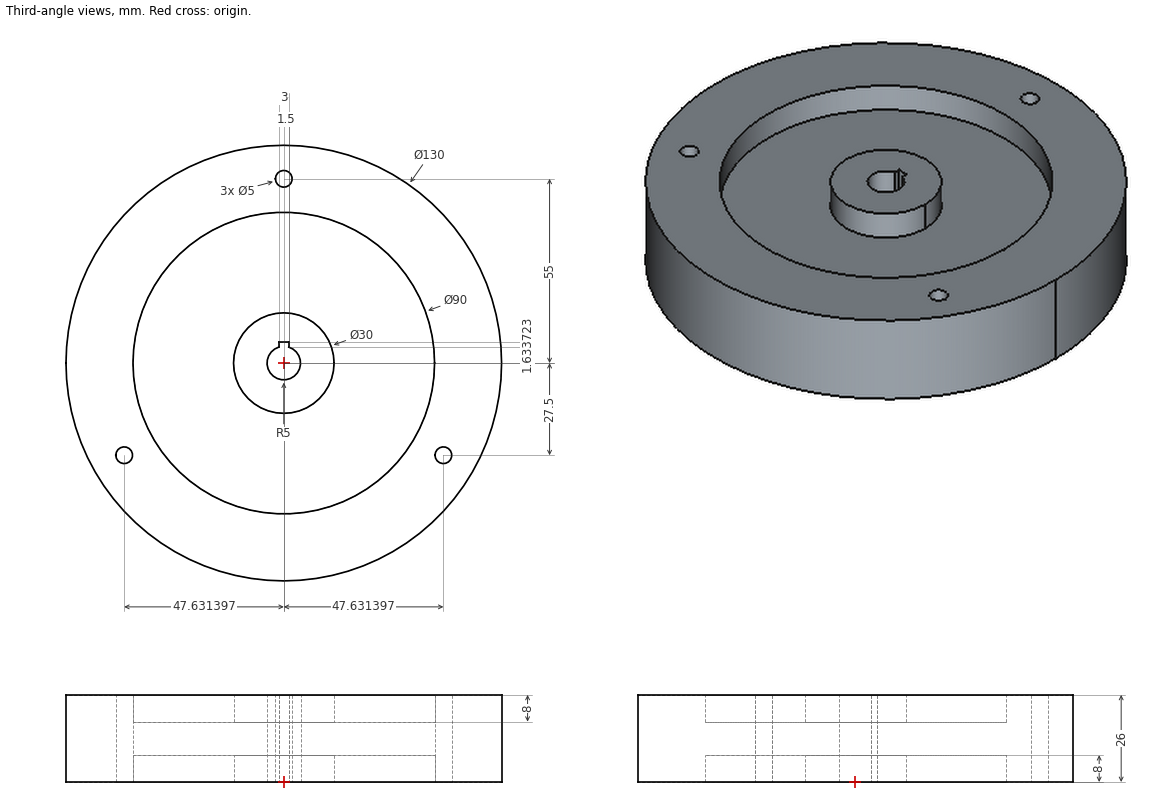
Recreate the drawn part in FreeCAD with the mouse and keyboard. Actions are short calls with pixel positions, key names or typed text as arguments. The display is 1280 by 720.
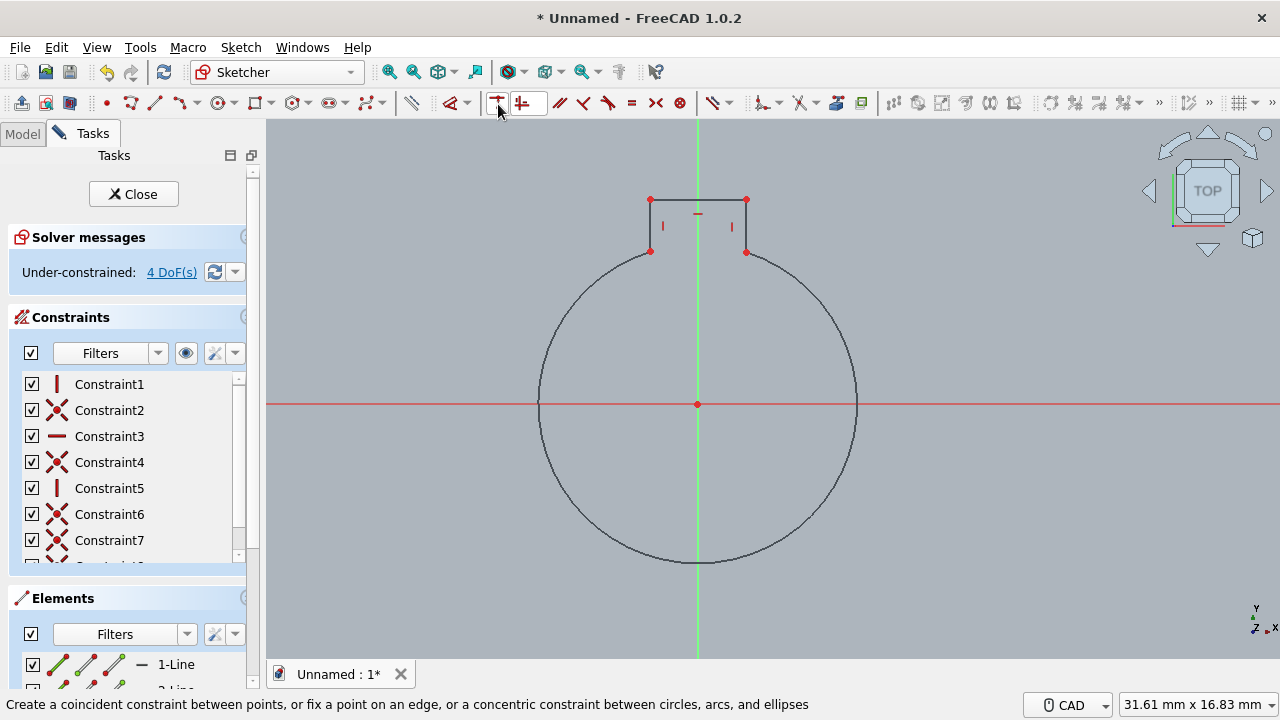
click(553, 471)
click(524, 484)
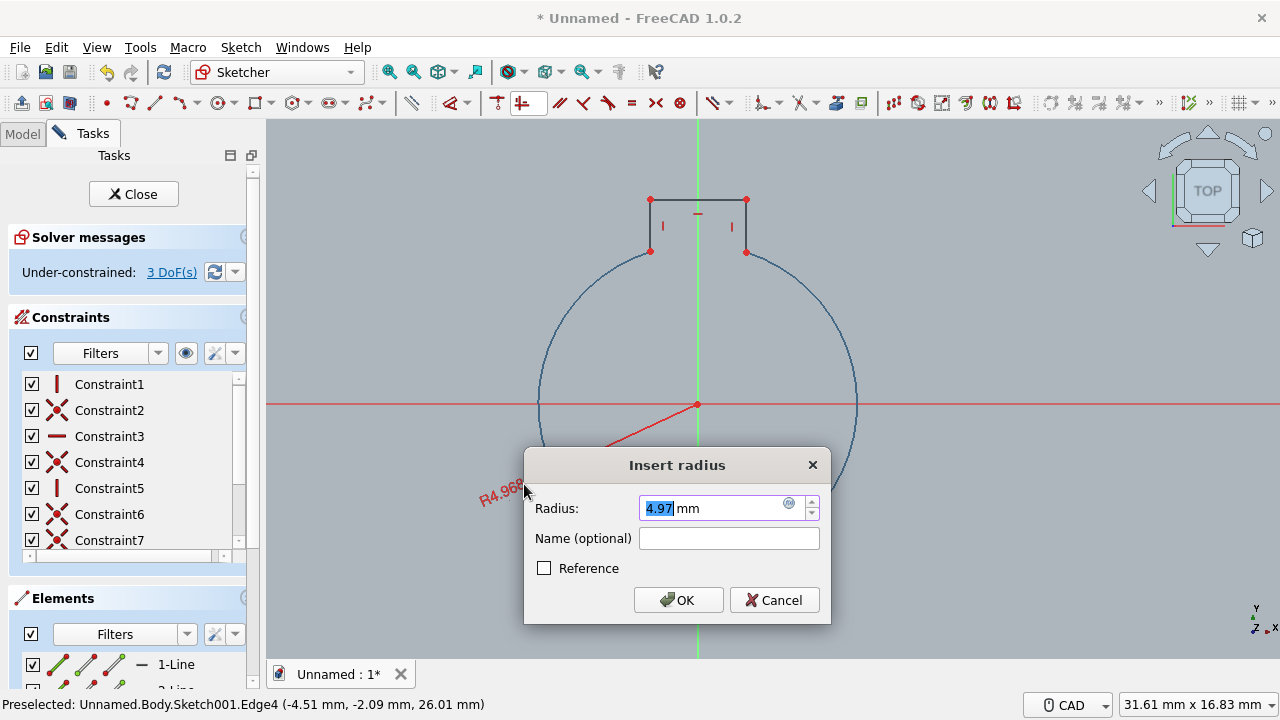
text(5)
key(Return)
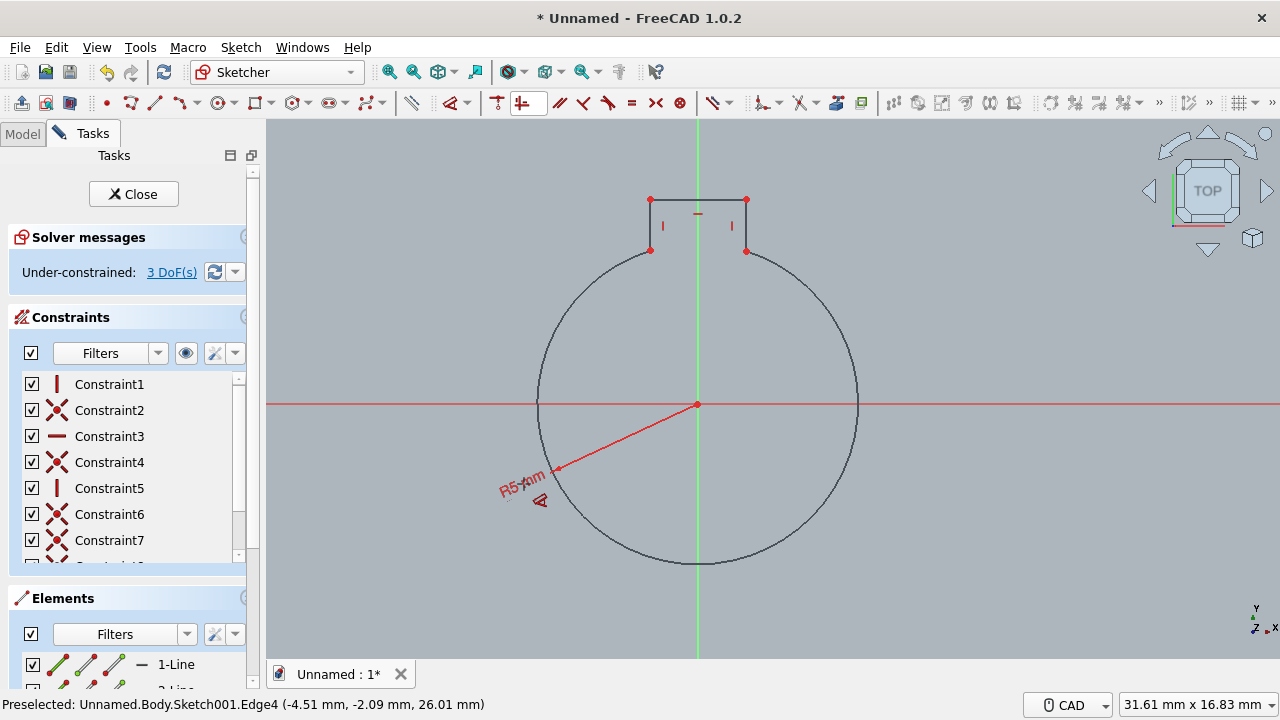
click(717, 200)
click(676, 166)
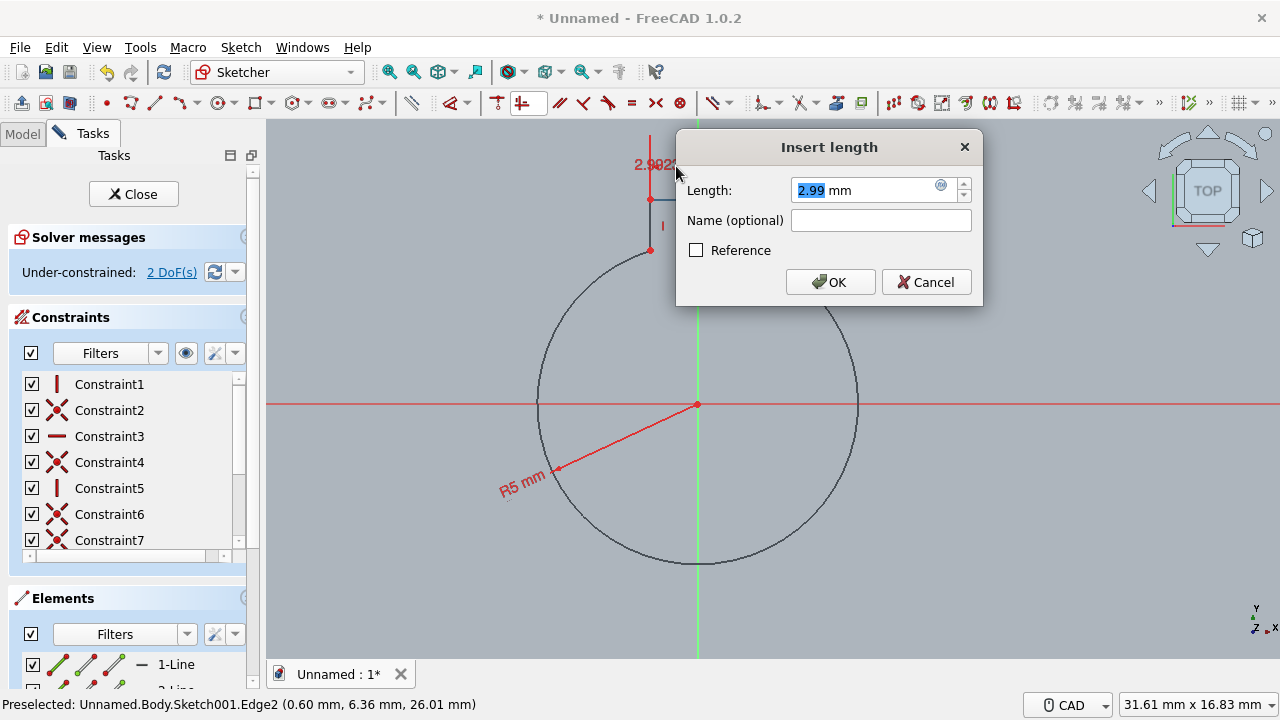
text(3)
key(Return)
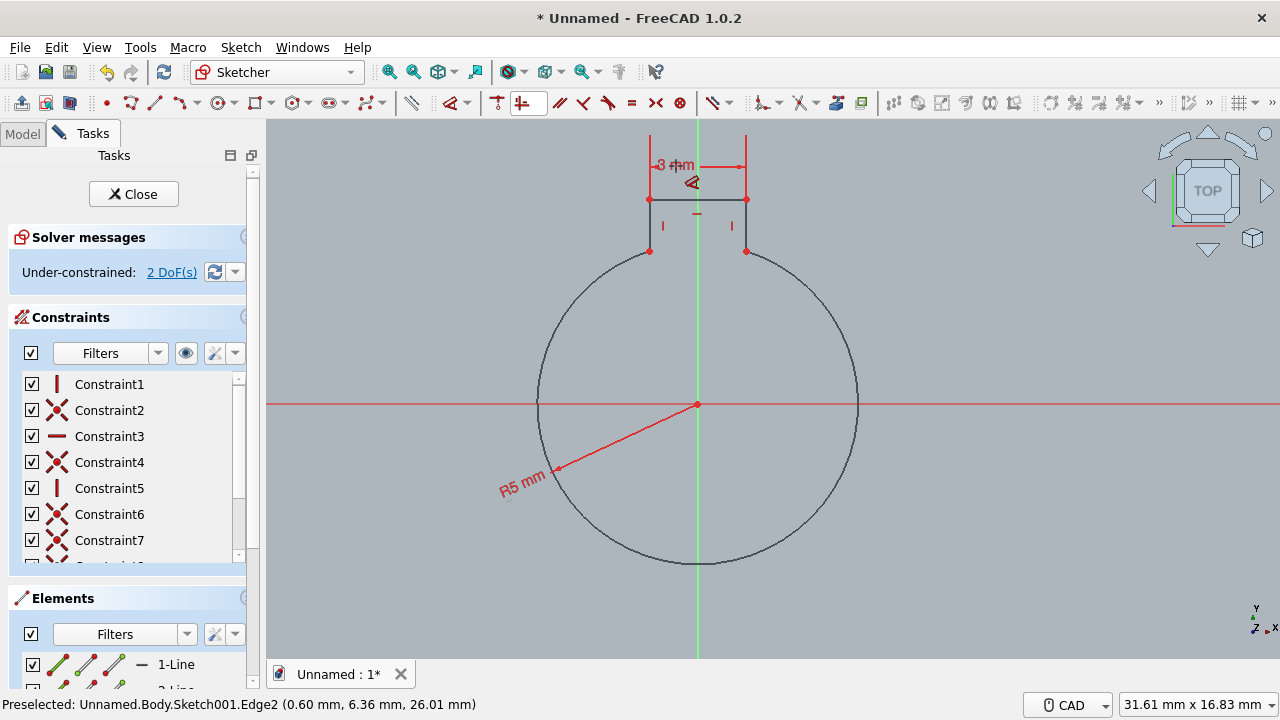
click(746, 251)
click(722, 217)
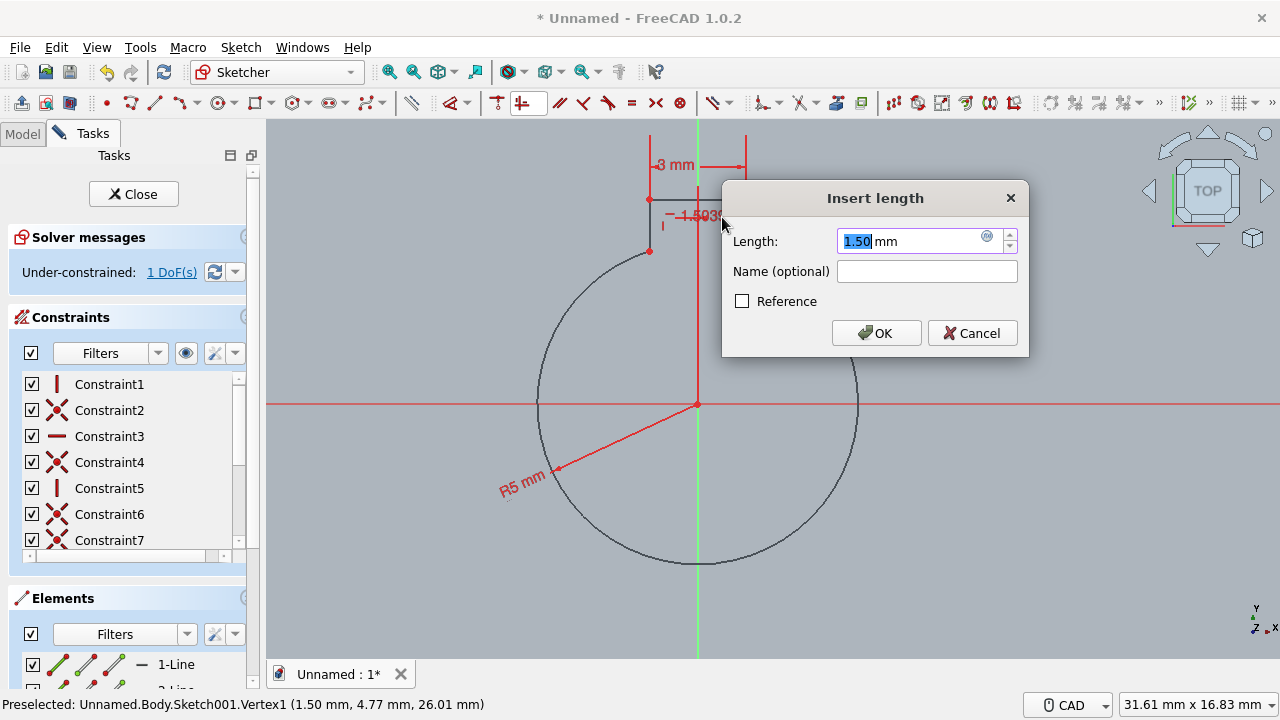
text(1.5)
key(Return)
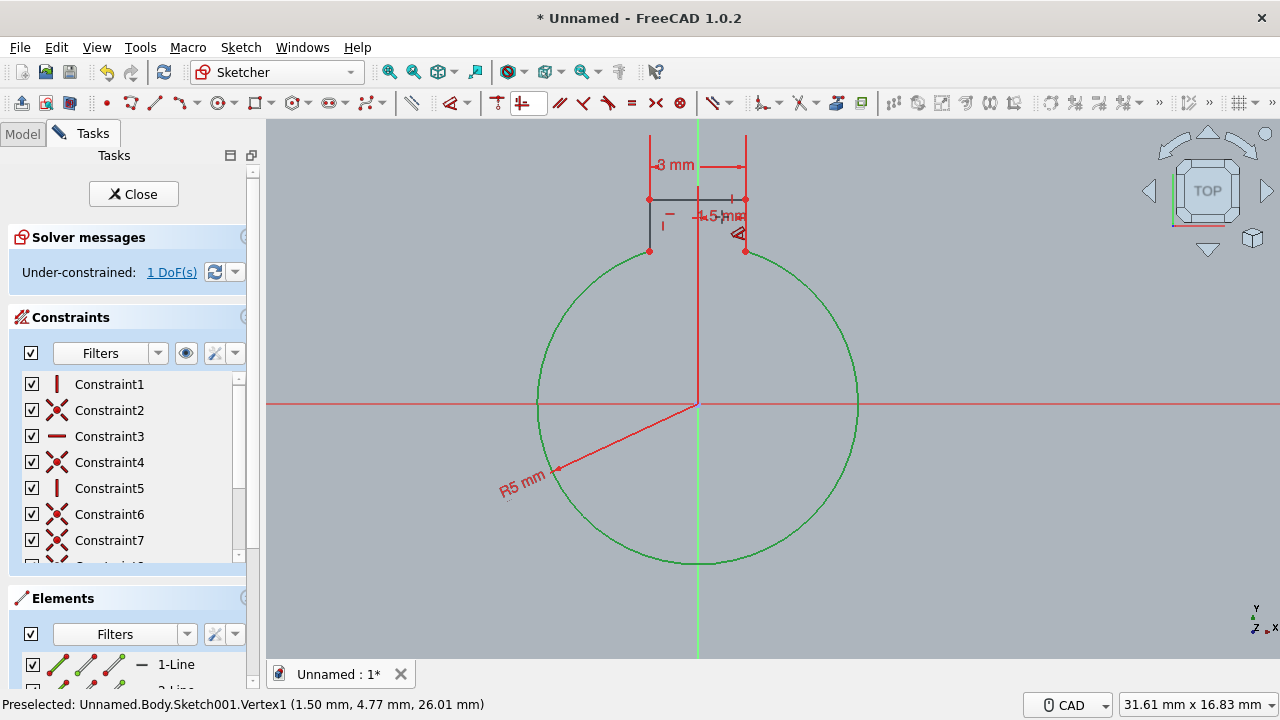
click(746, 236)
click(780, 237)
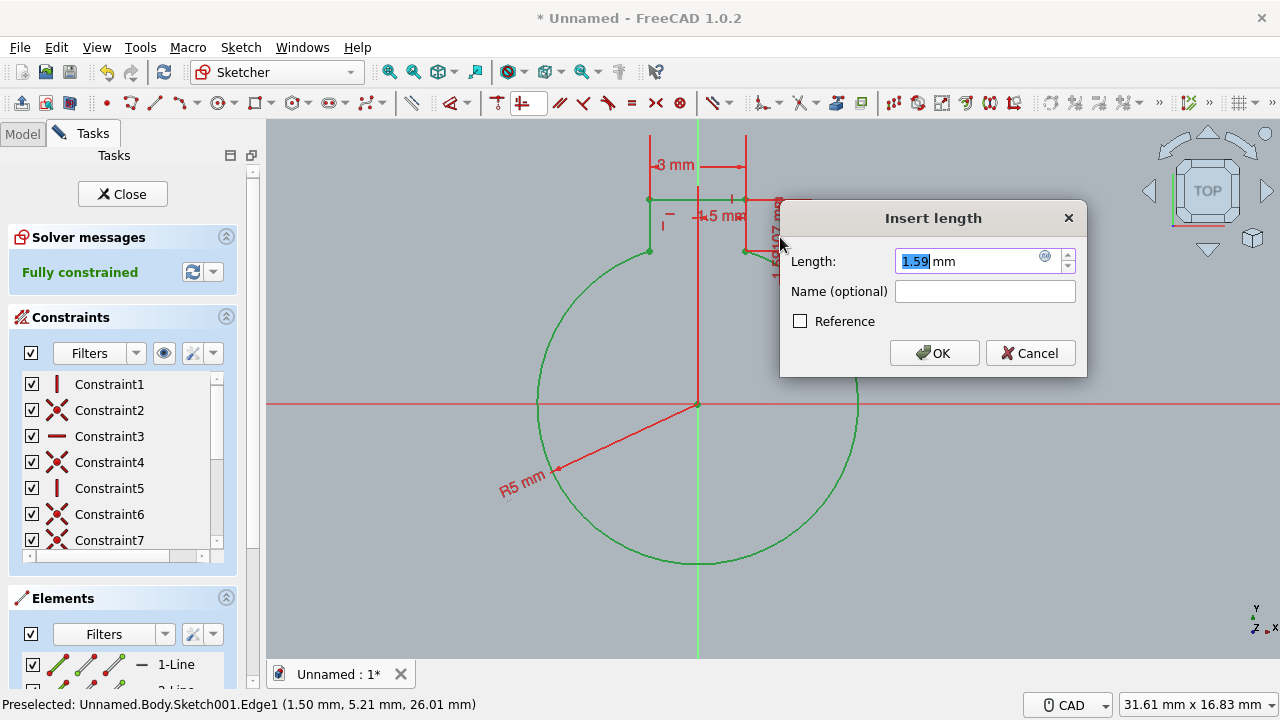
text(1.633723)
key(Return)
key(Escape)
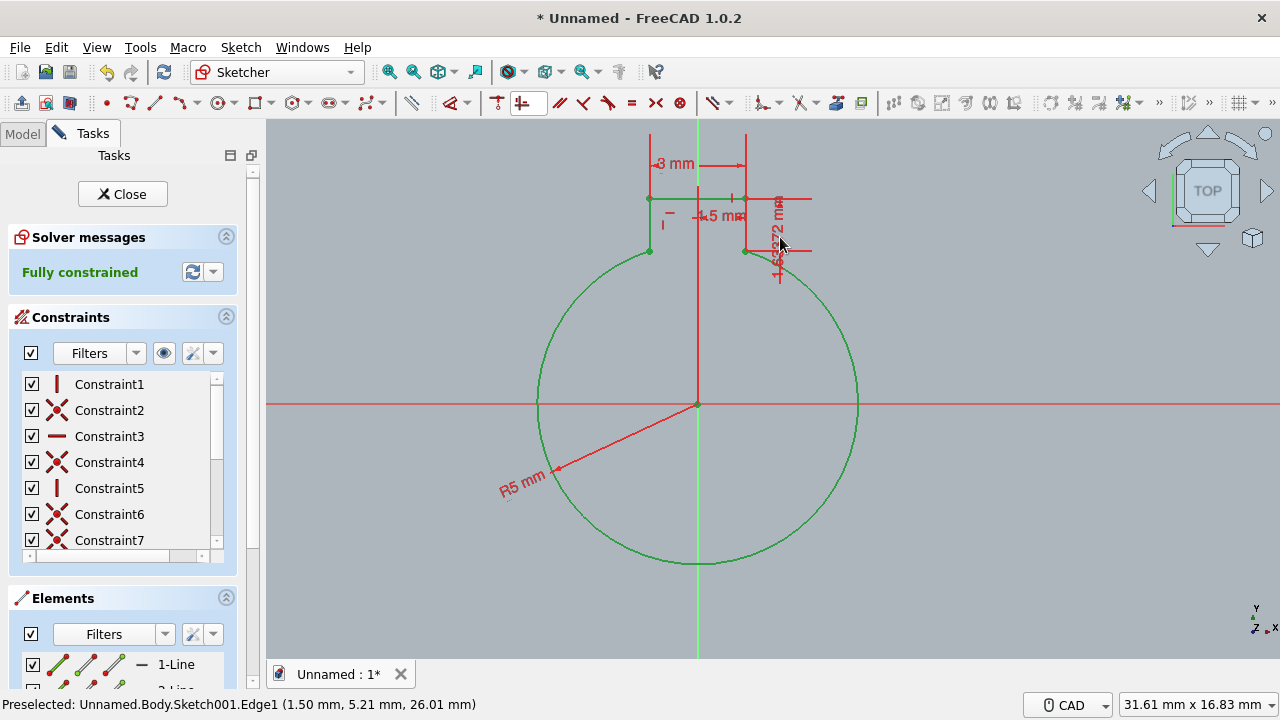
click(123, 194)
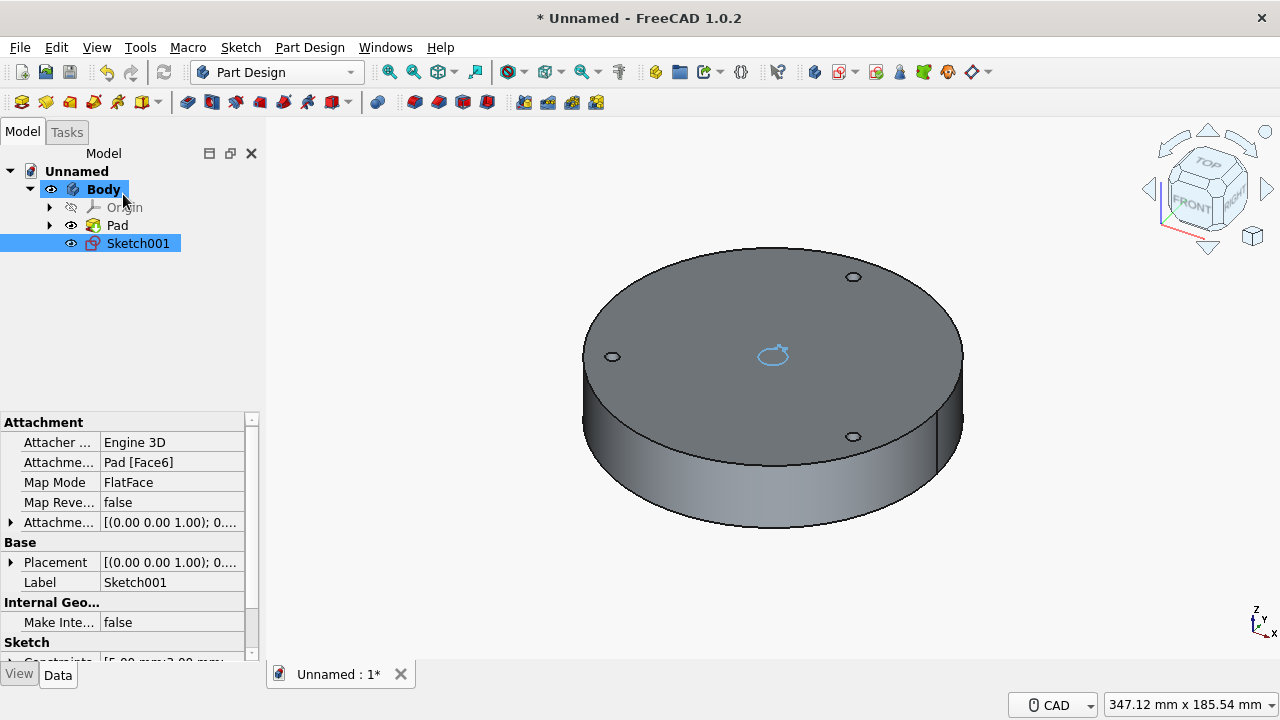
click(188, 102)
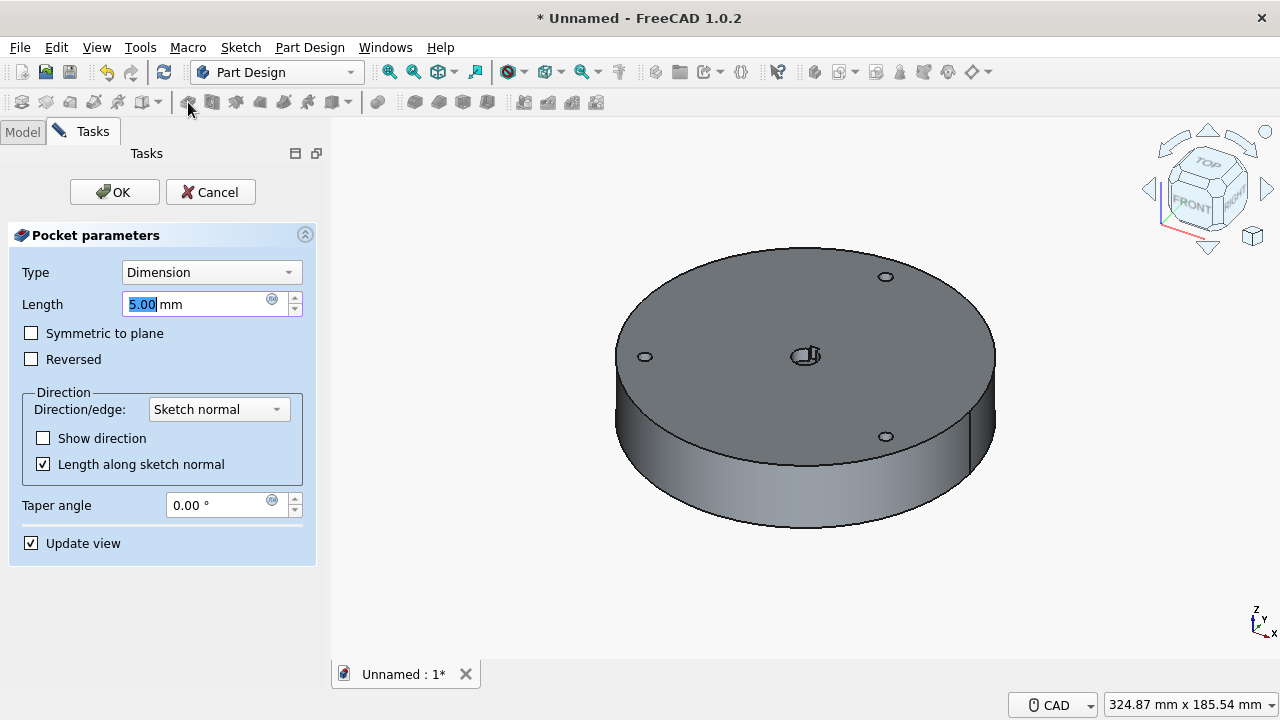
click(212, 272)